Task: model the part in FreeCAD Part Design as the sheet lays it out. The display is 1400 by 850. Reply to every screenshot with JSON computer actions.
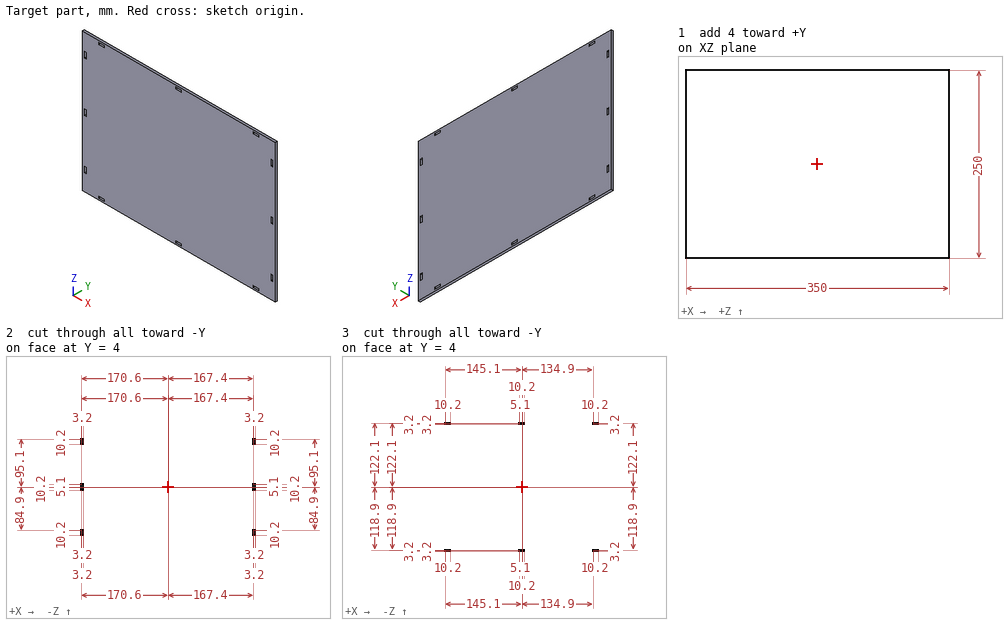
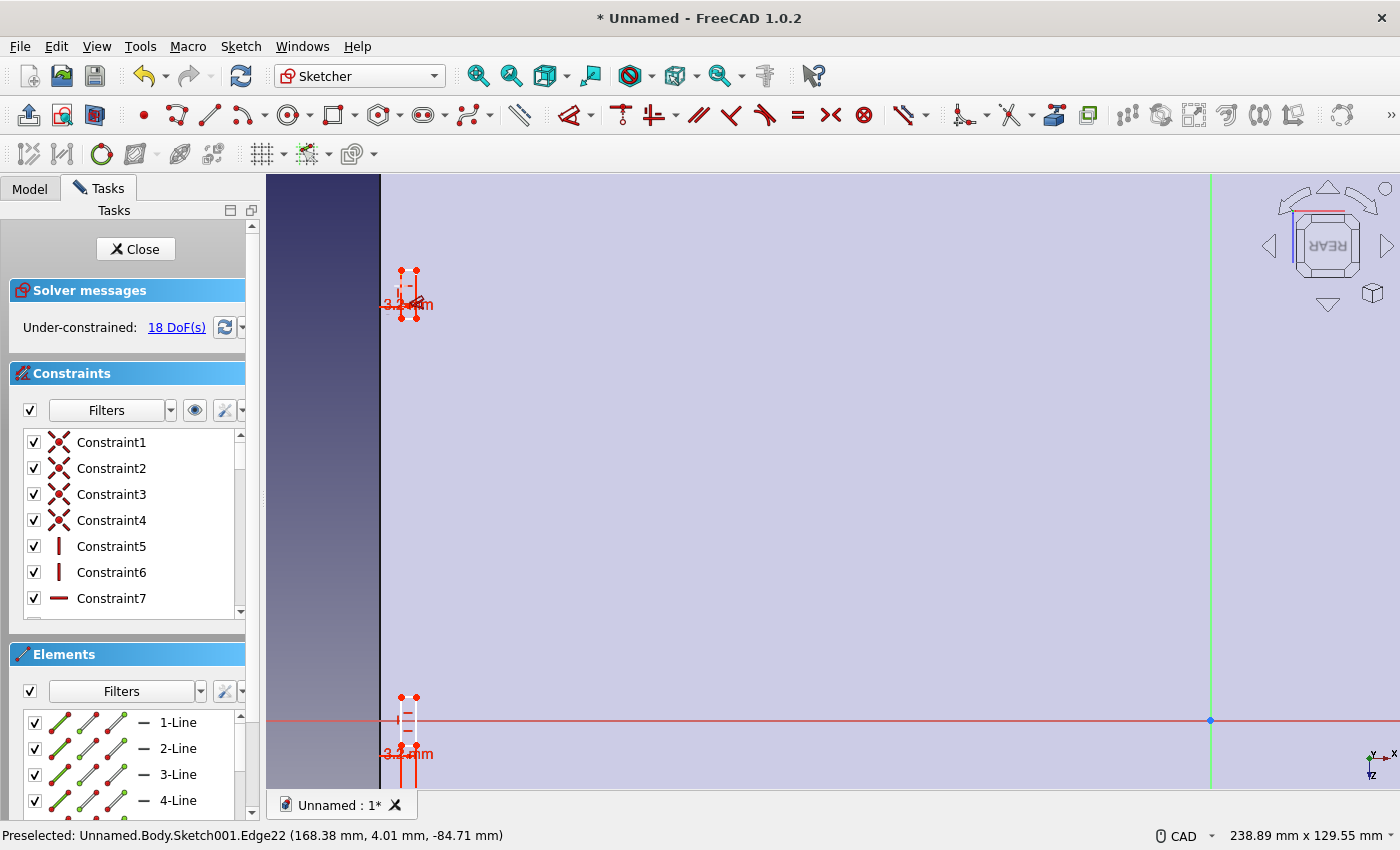
{"action": "left_click", "coordinate": [401, 285]}
{"action": "left_click", "coordinate": [367, 283]}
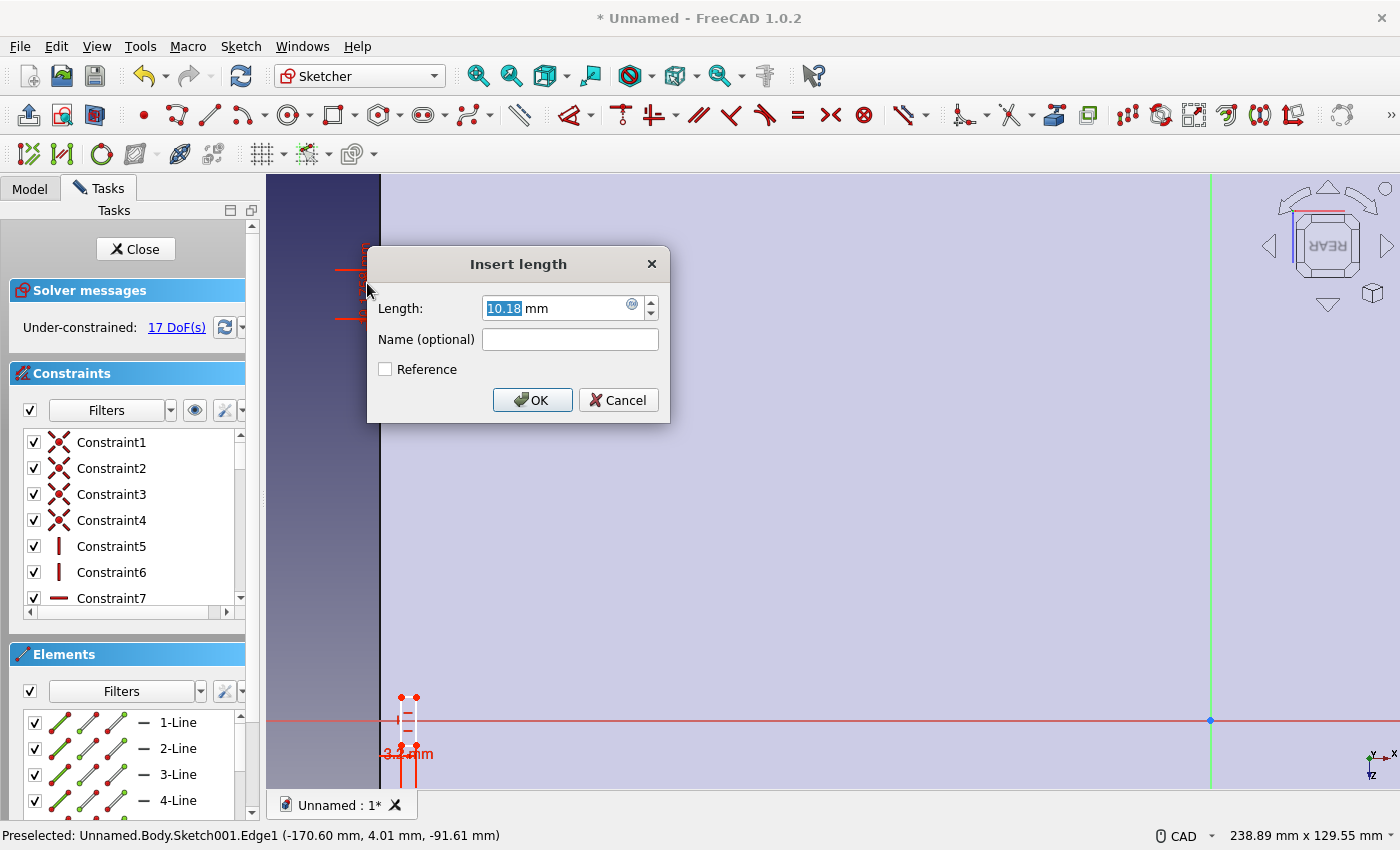
{"action": "type", "text": "10.2"}
{"action": "key", "text": "Return"}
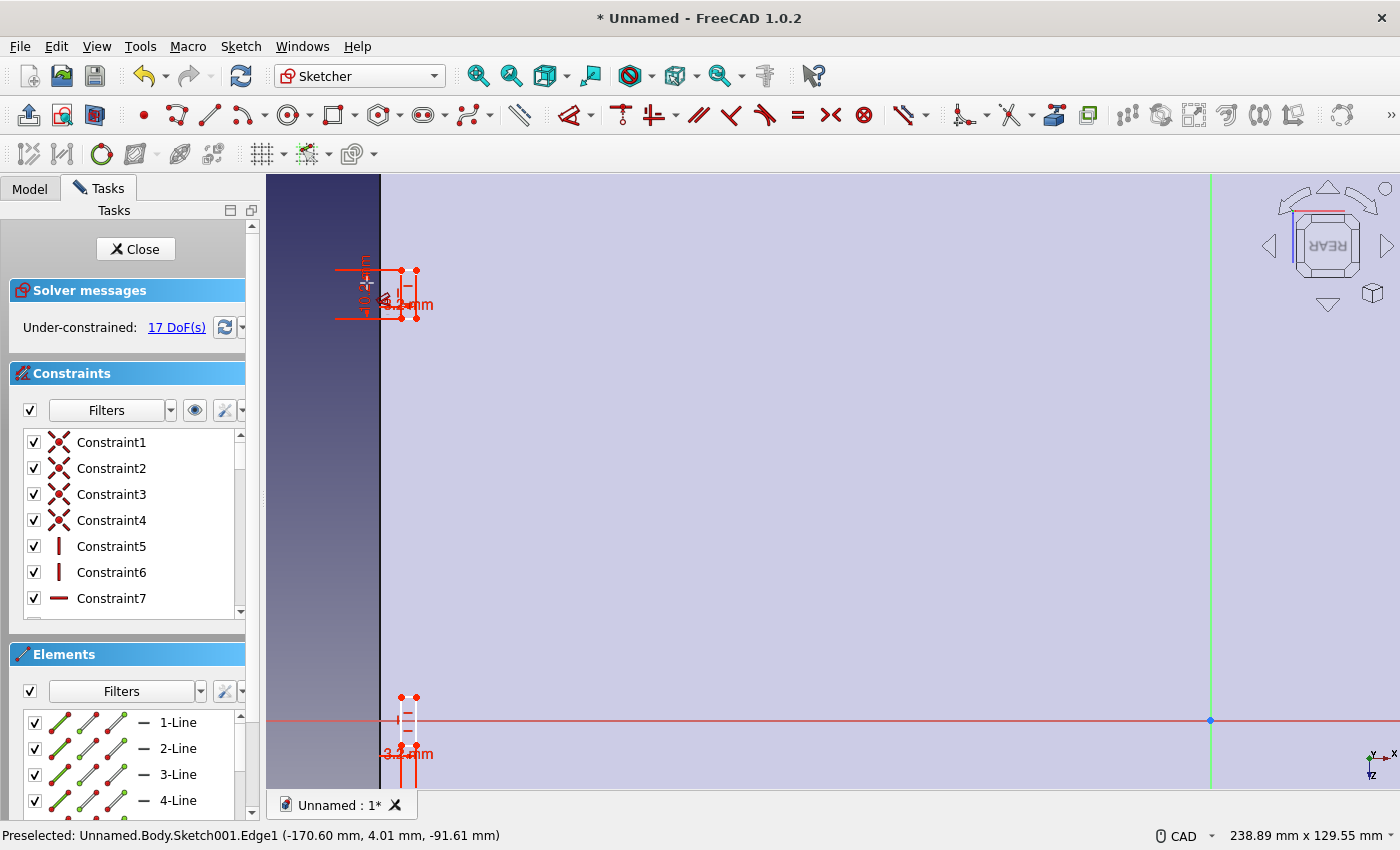
{"action": "scroll", "coordinate": [401, 712], "scroll_direction": "up", "scroll_amount": 3}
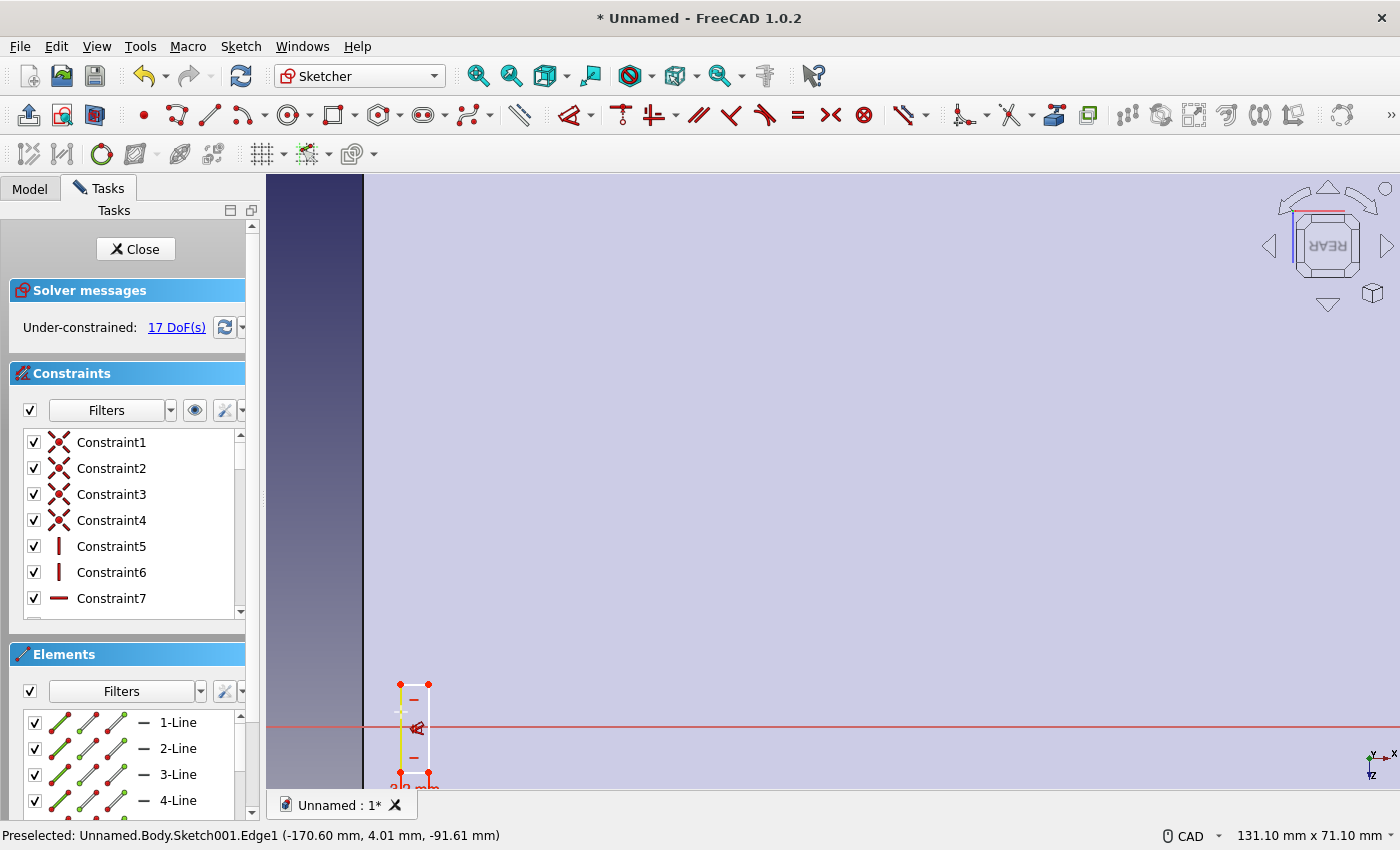
{"action": "left_click", "coordinate": [401, 711]}
{"action": "left_click", "coordinate": [367, 705]}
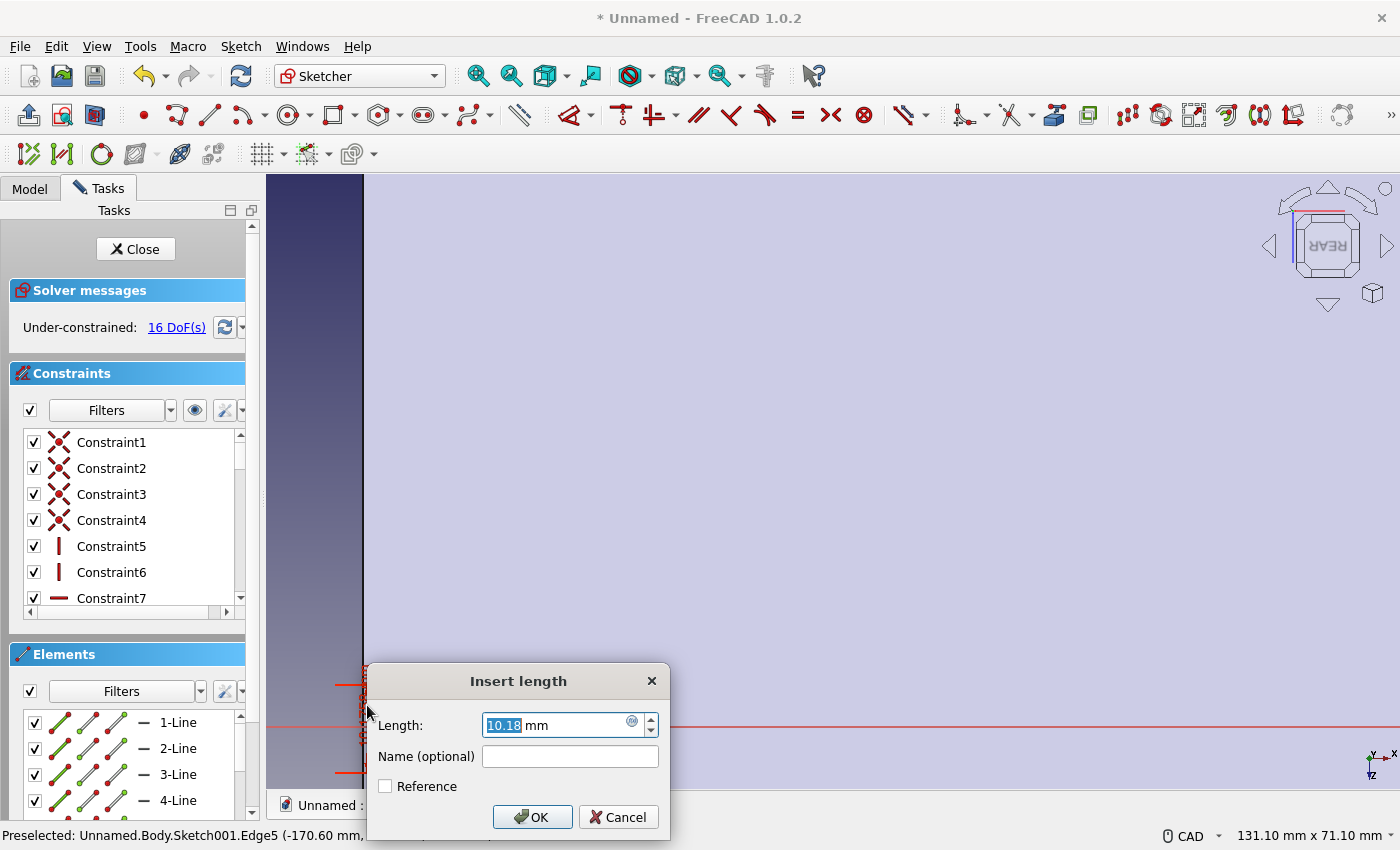
{"action": "type", "text": "10.2"}
{"action": "key", "text": "Return"}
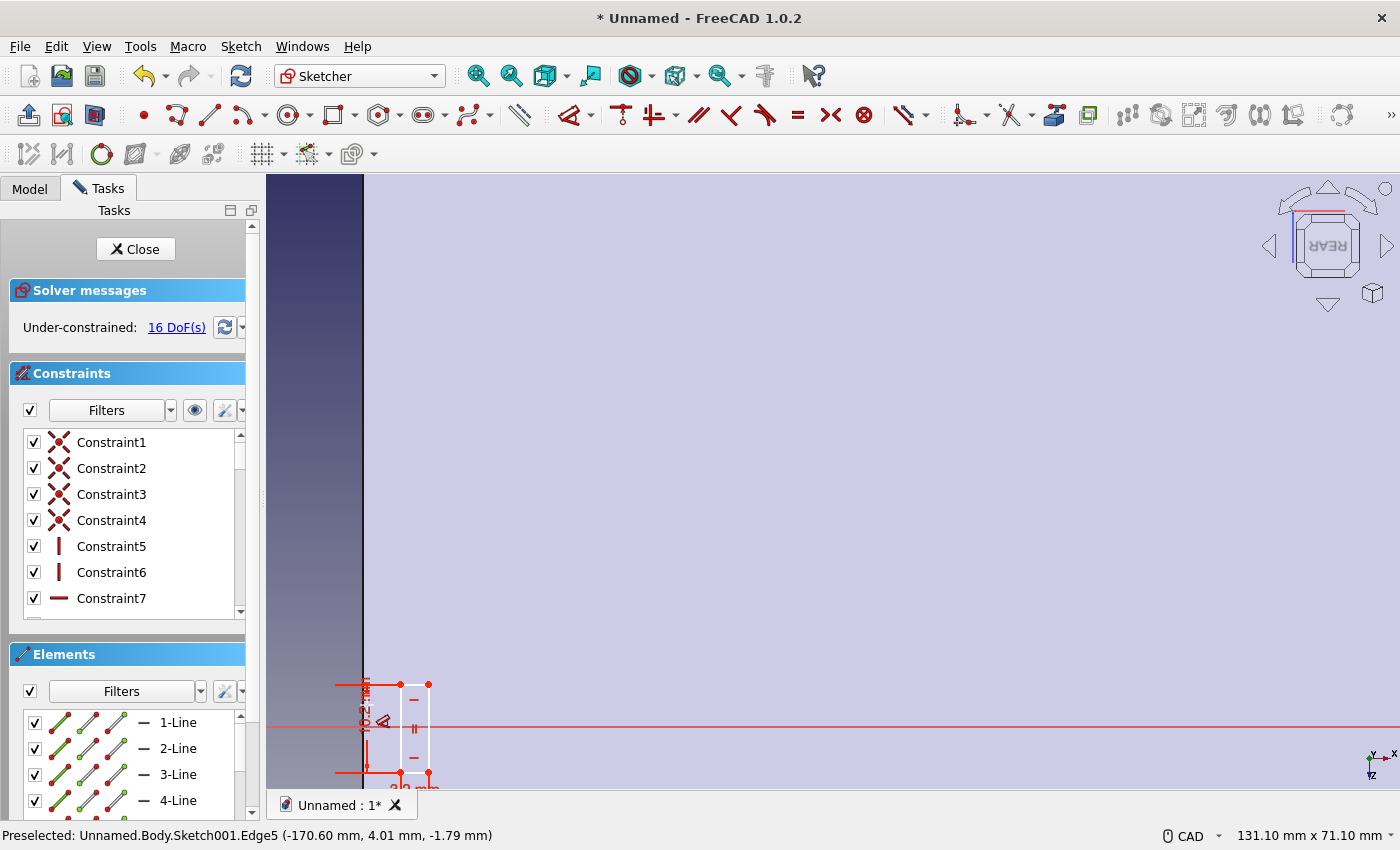
{"action": "scroll", "coordinate": [401, 401], "scroll_direction": "down", "scroll_amount": 7}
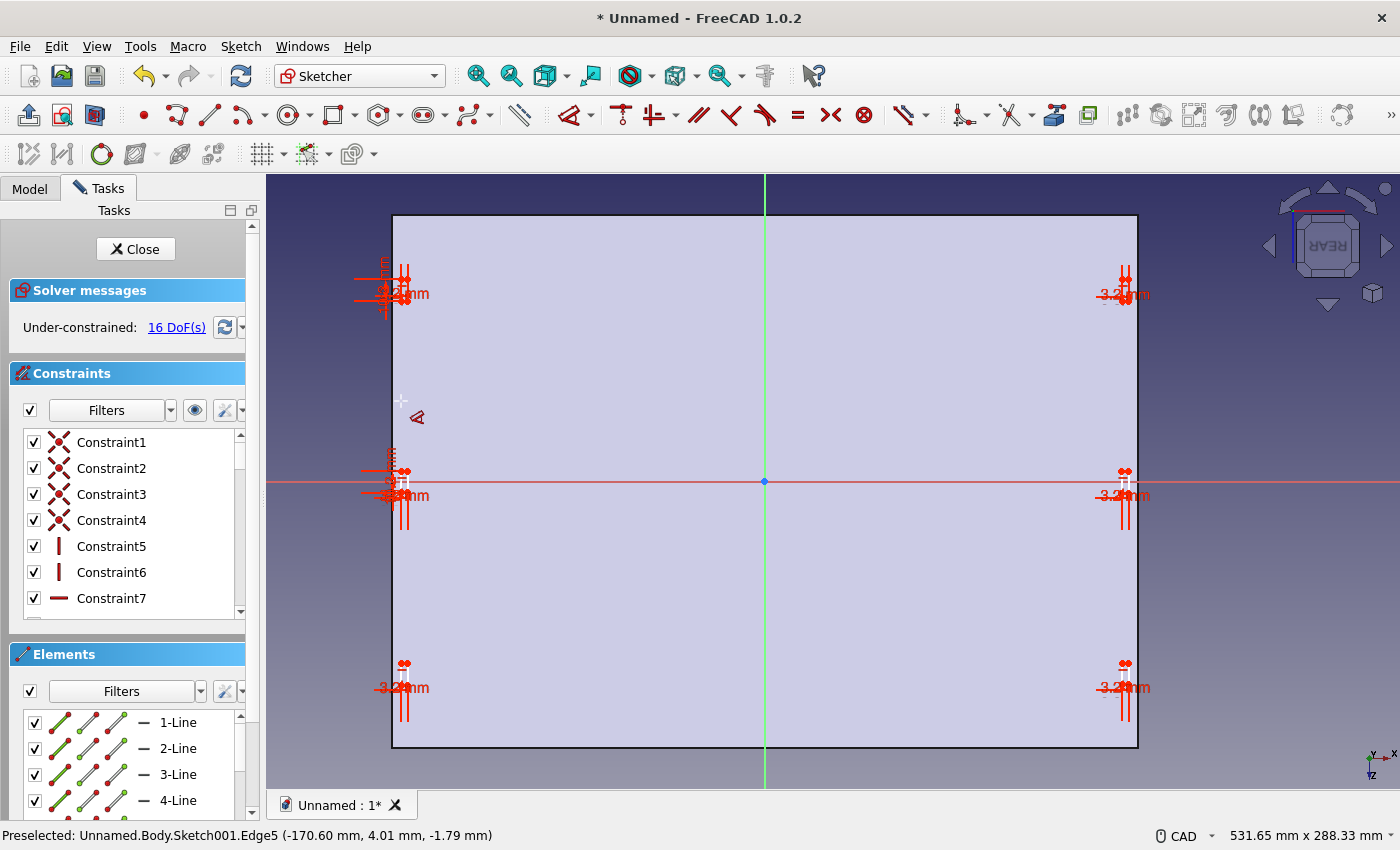
{"action": "scroll", "coordinate": [401, 670], "scroll_direction": "up", "scroll_amount": 4}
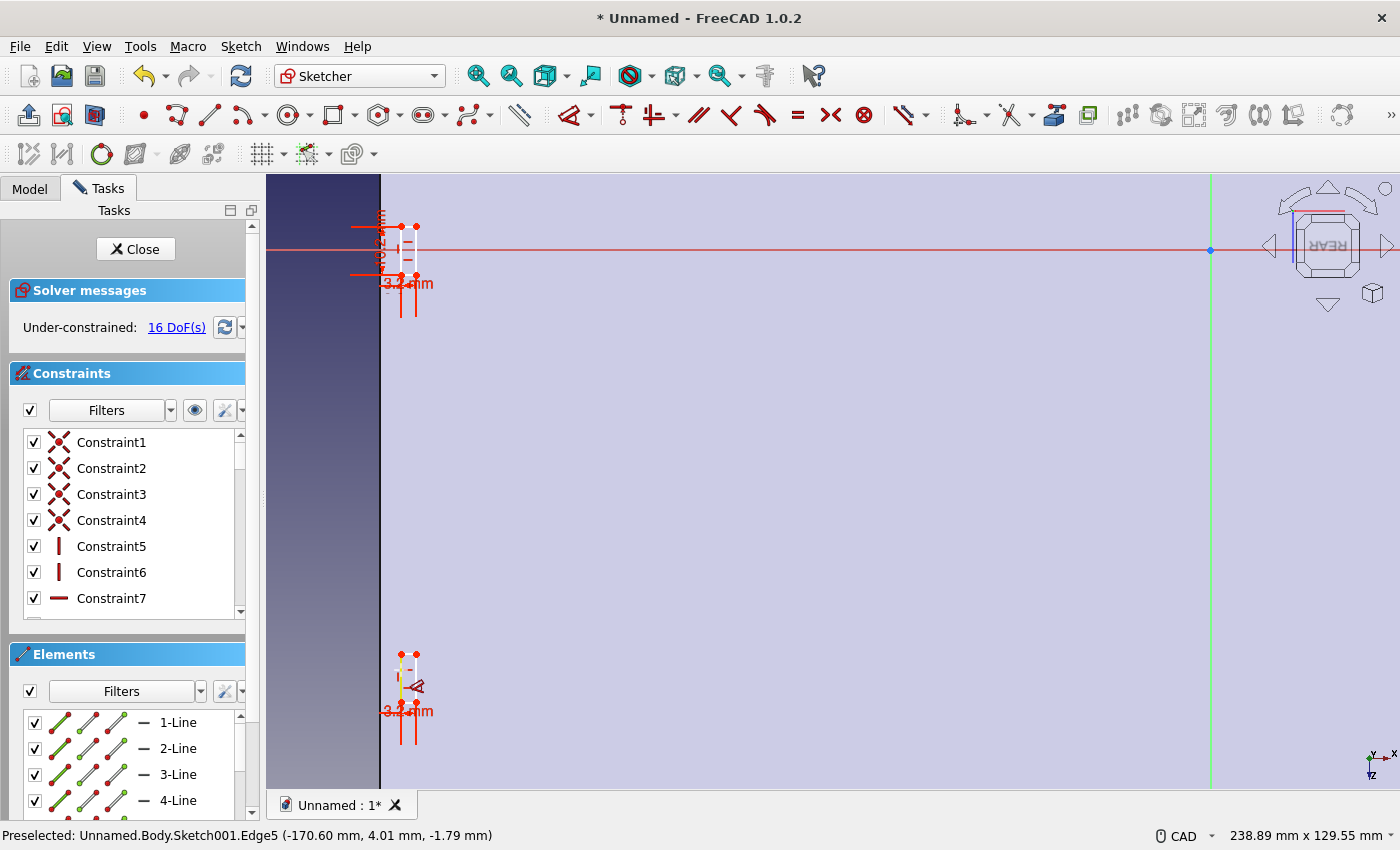
{"action": "left_click", "coordinate": [401, 669]}
{"action": "left_click", "coordinate": [367, 679]}